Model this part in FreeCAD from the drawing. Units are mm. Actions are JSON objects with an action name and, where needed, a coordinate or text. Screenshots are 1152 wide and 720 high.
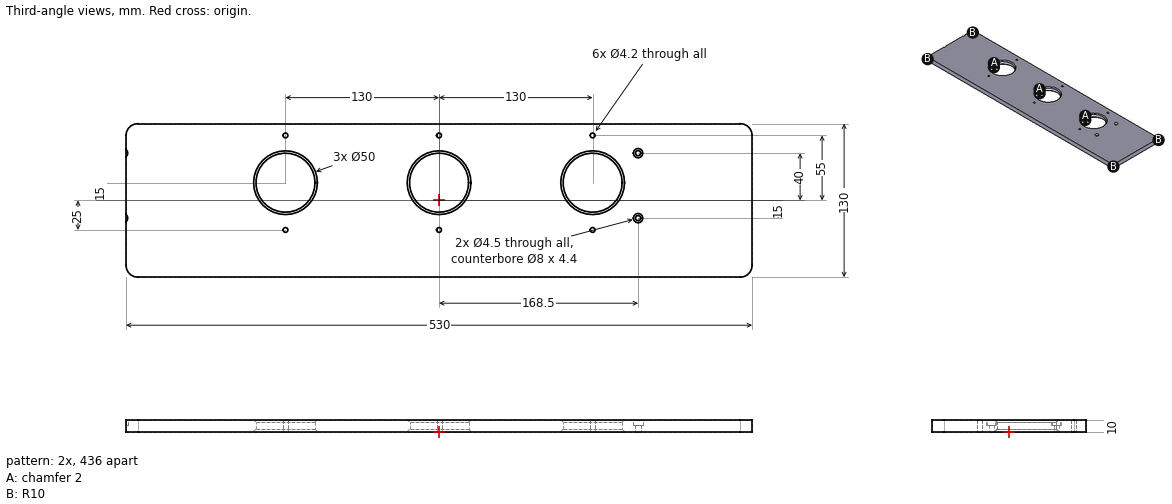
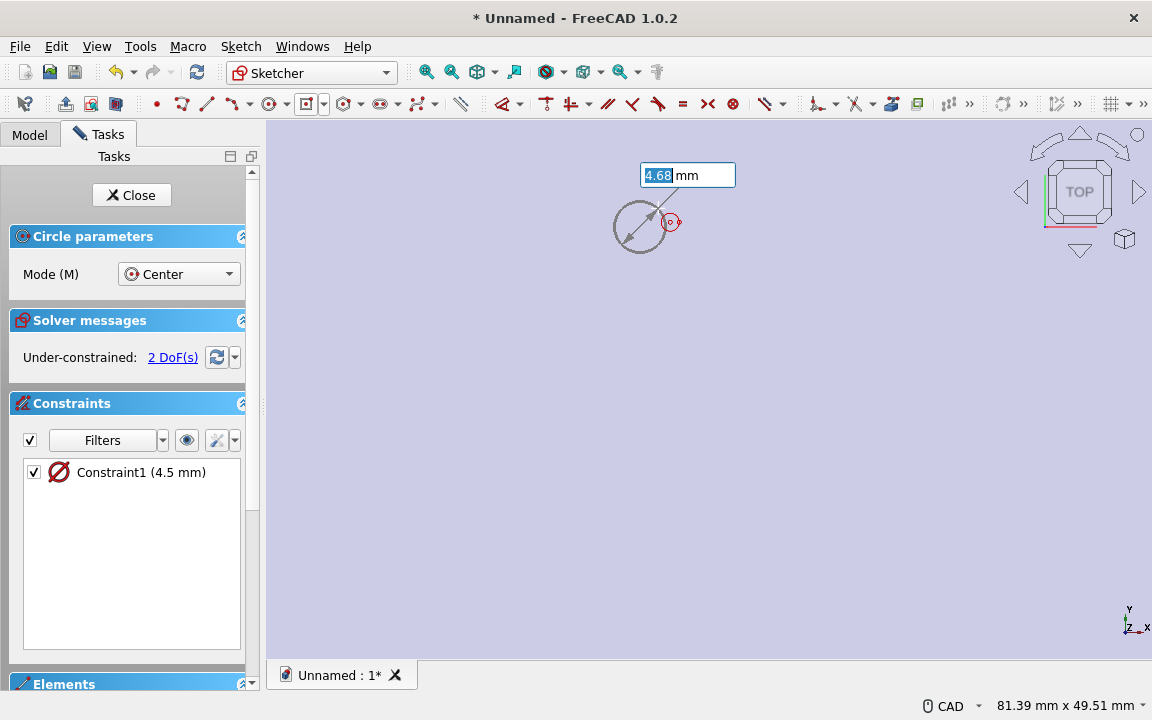
{"action": "type", "text": "4.5"}
{"action": "key", "text": "Return"}
{"action": "key", "text": "Escape"}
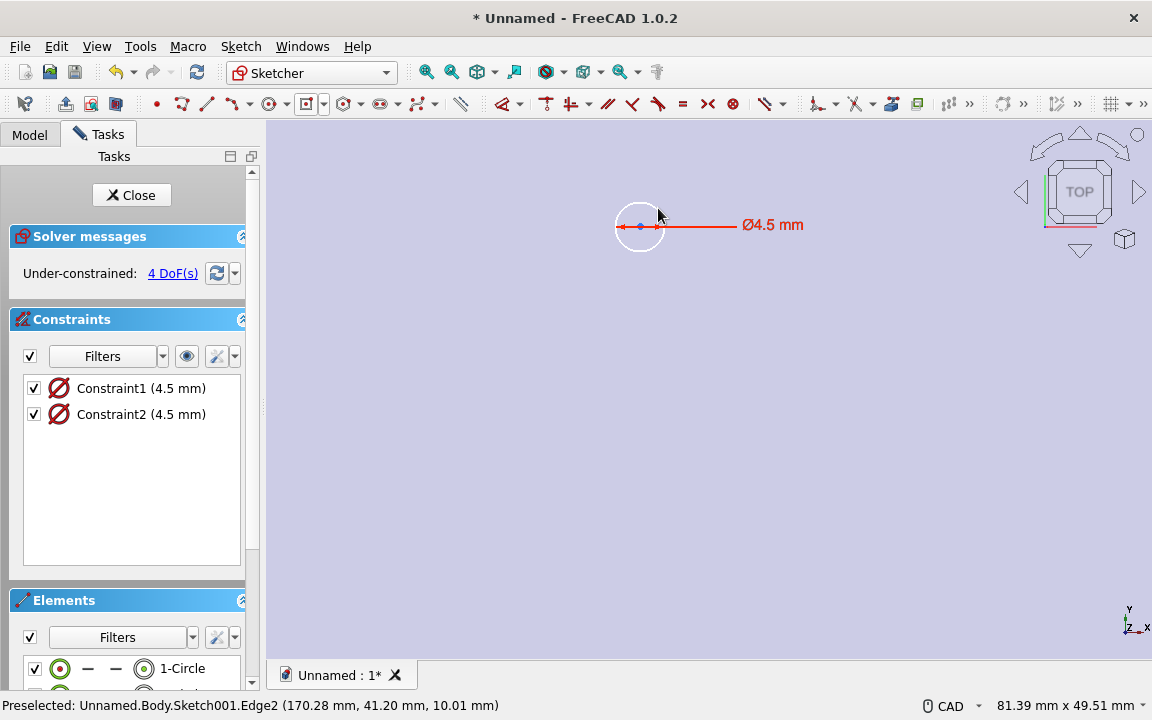
{"action": "scroll", "coordinate": [641, 225], "scroll_direction": "down", "scroll_amount": 3}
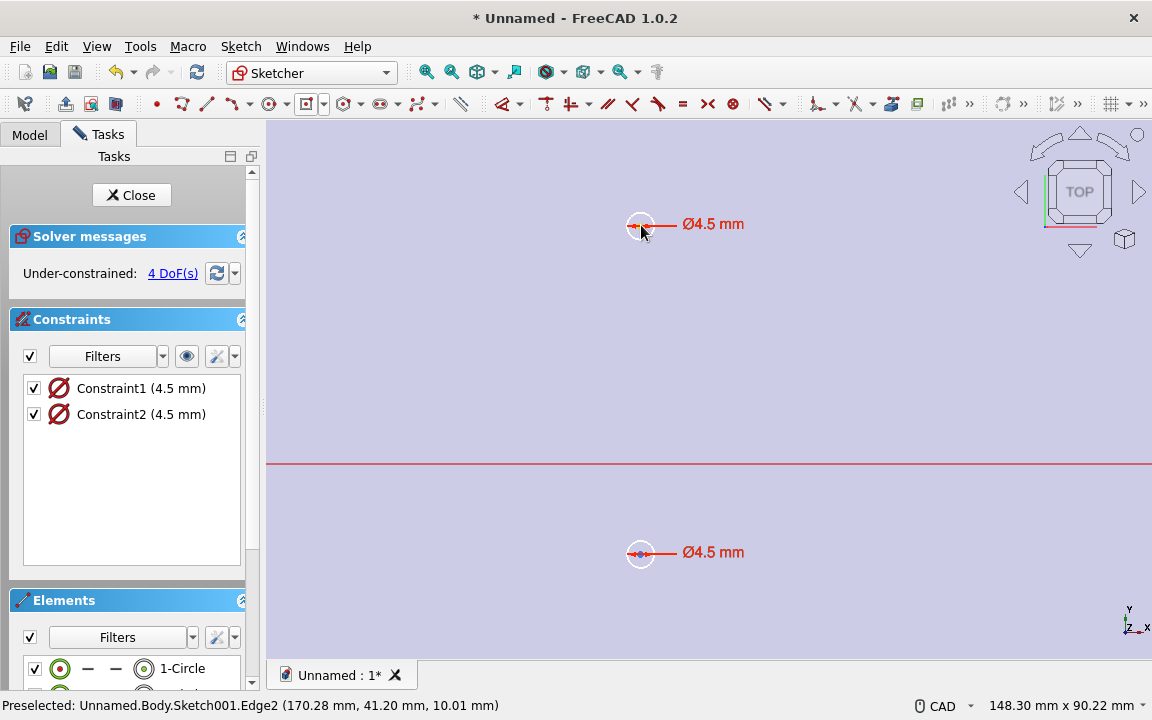
{"action": "left_click", "coordinate": [641, 554]}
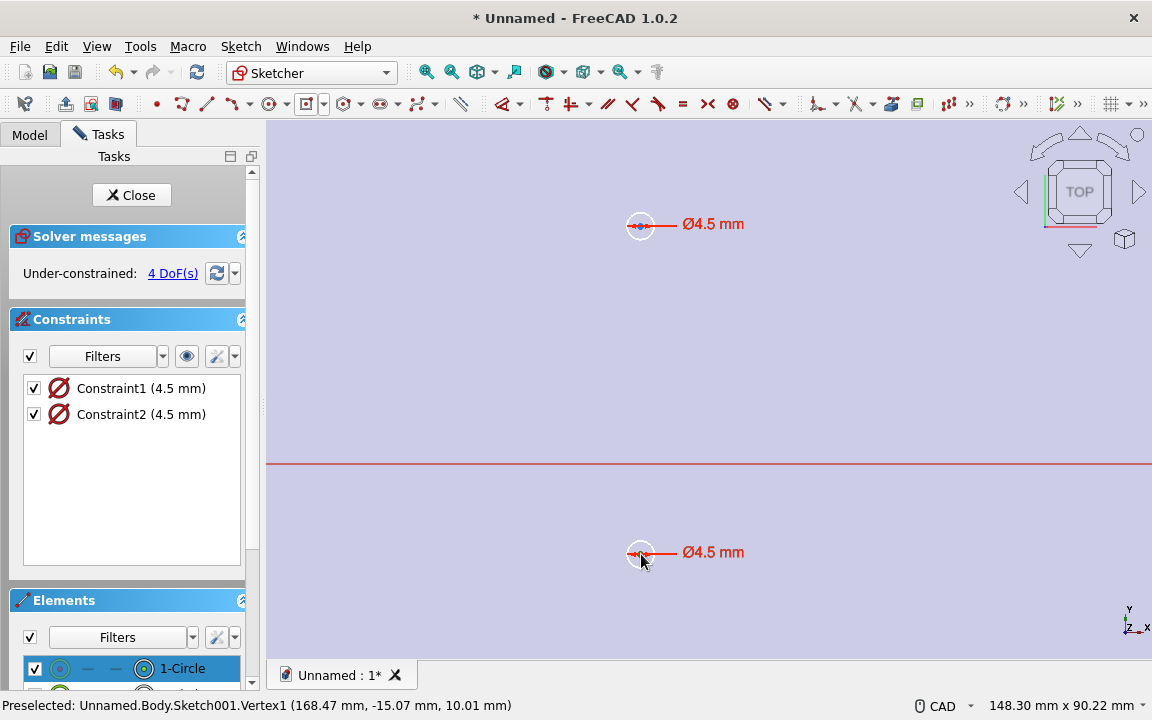
{"action": "left_click", "coordinate": [641, 226]}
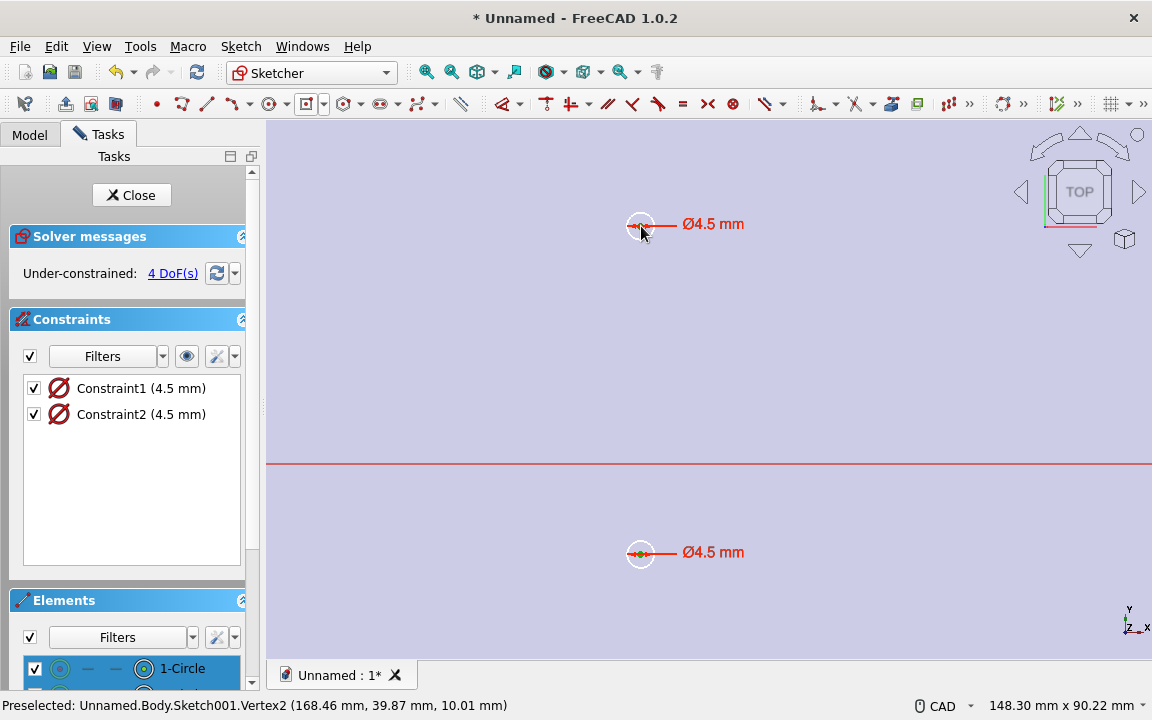
{"action": "key", "text": "v"}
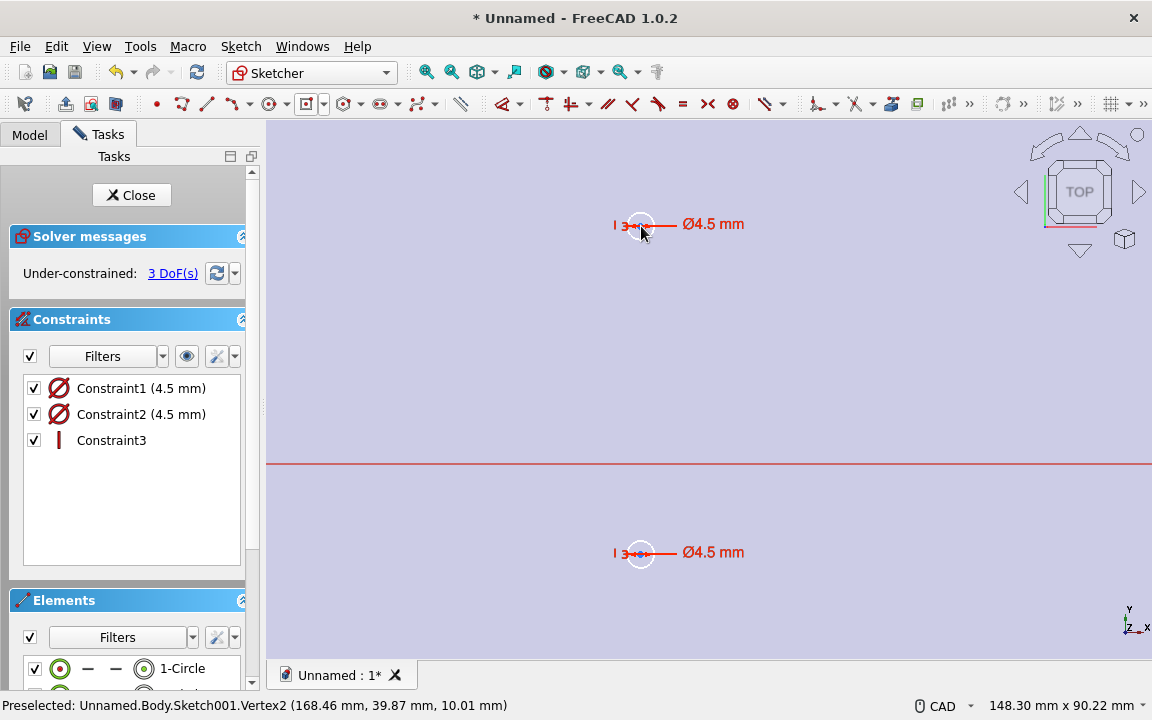
{"action": "left_click", "coordinate": [502, 104]}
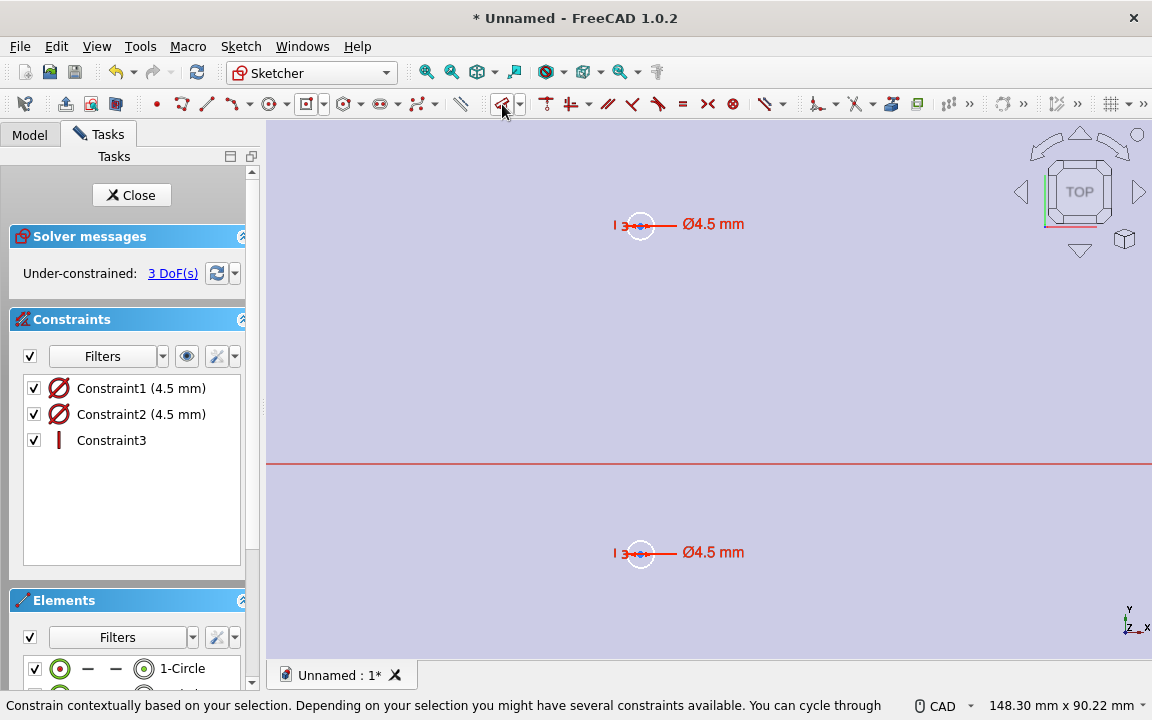
{"action": "left_click", "coordinate": [641, 554]}
{"action": "left_click", "coordinate": [675, 509]}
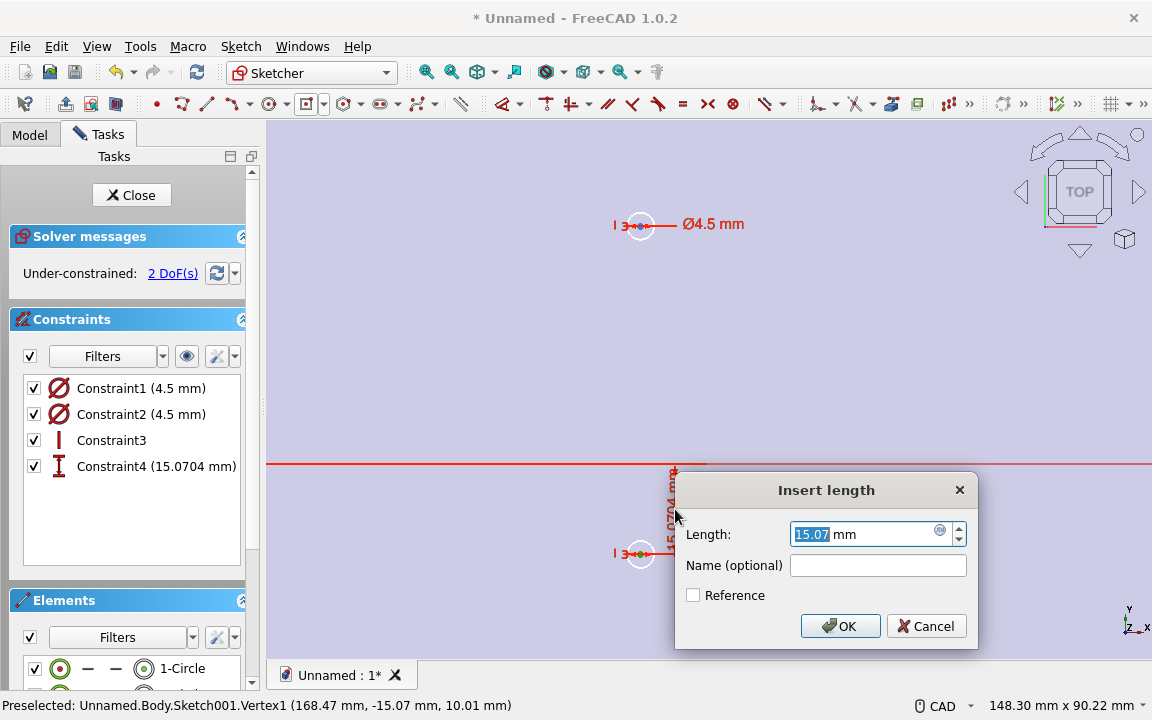
{"action": "type", "text": "15"}
{"action": "key", "text": "Return"}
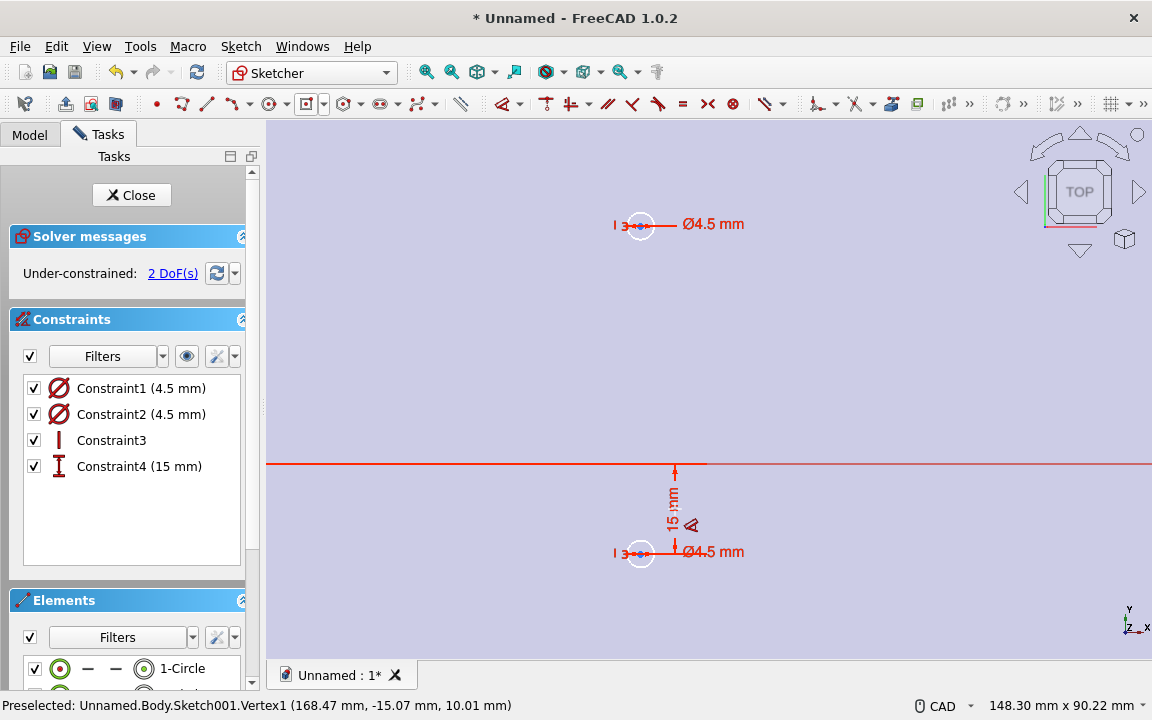
{"action": "left_click", "coordinate": [641, 226]}
{"action": "left_click", "coordinate": [675, 345]}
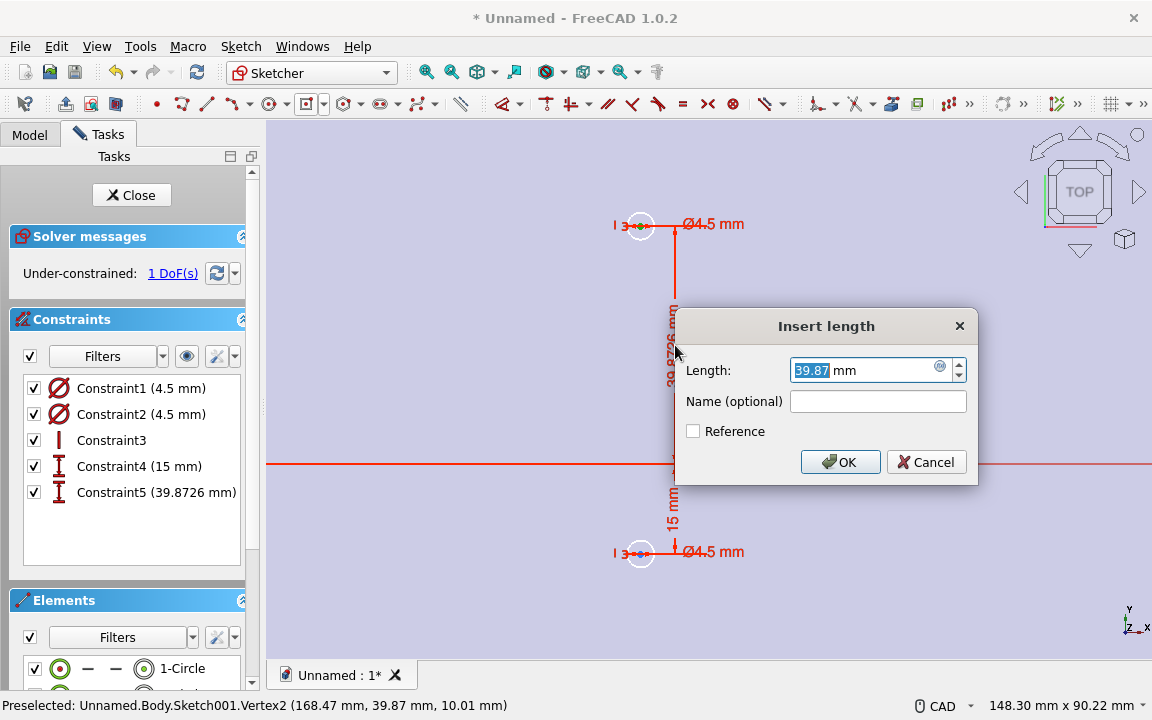
{"action": "type", "text": "40"}
{"action": "key", "text": "Return"}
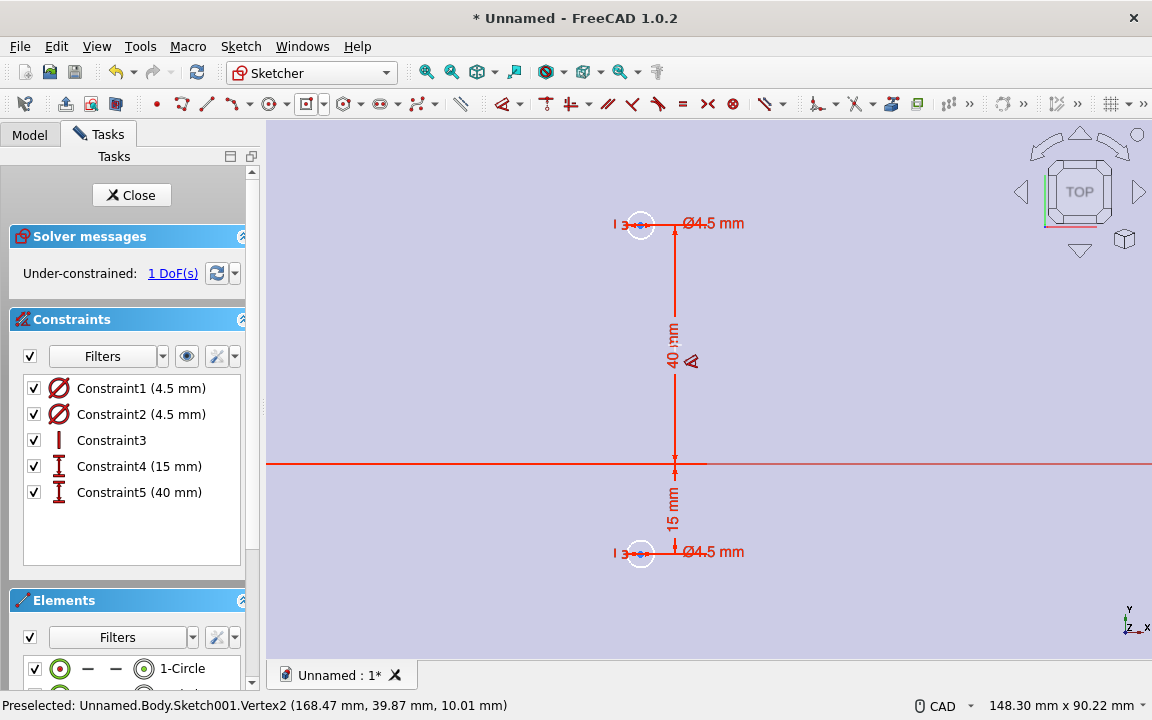
{"action": "left_click", "coordinate": [641, 554]}
{"action": "left_click", "coordinate": [467, 588]}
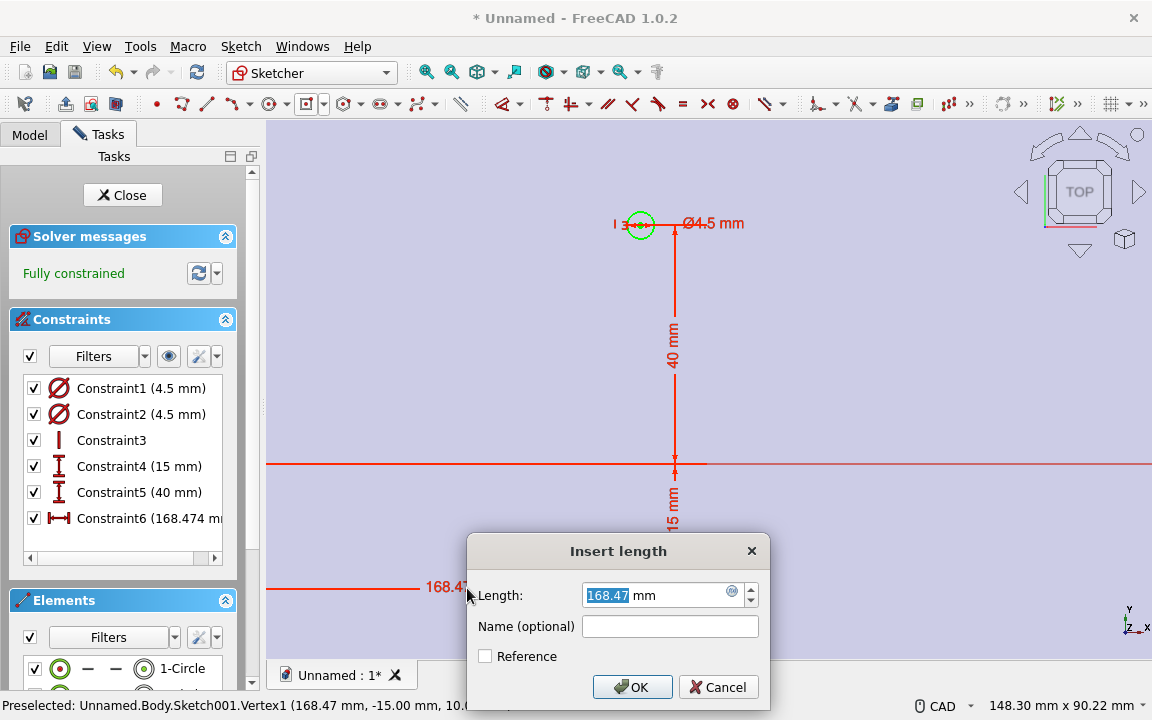
{"action": "type", "text": "168.5"}
{"action": "key", "text": "Return"}
{"action": "key", "text": "Escape"}